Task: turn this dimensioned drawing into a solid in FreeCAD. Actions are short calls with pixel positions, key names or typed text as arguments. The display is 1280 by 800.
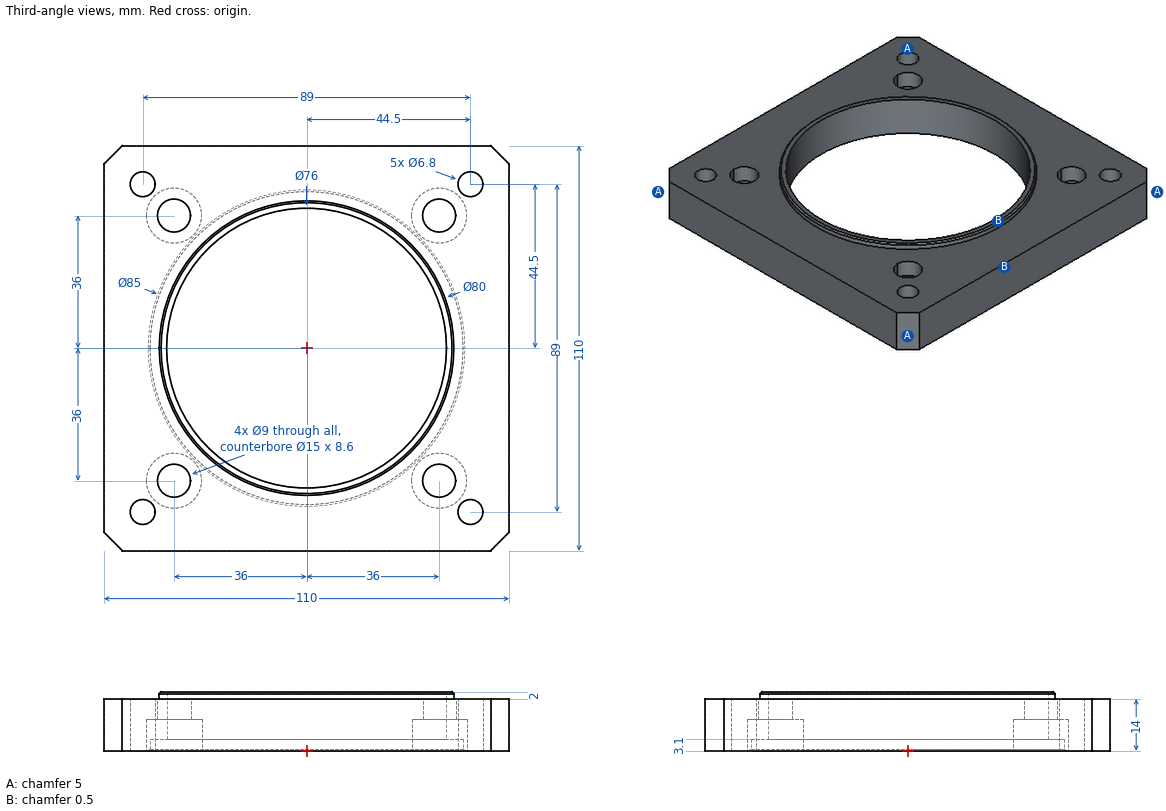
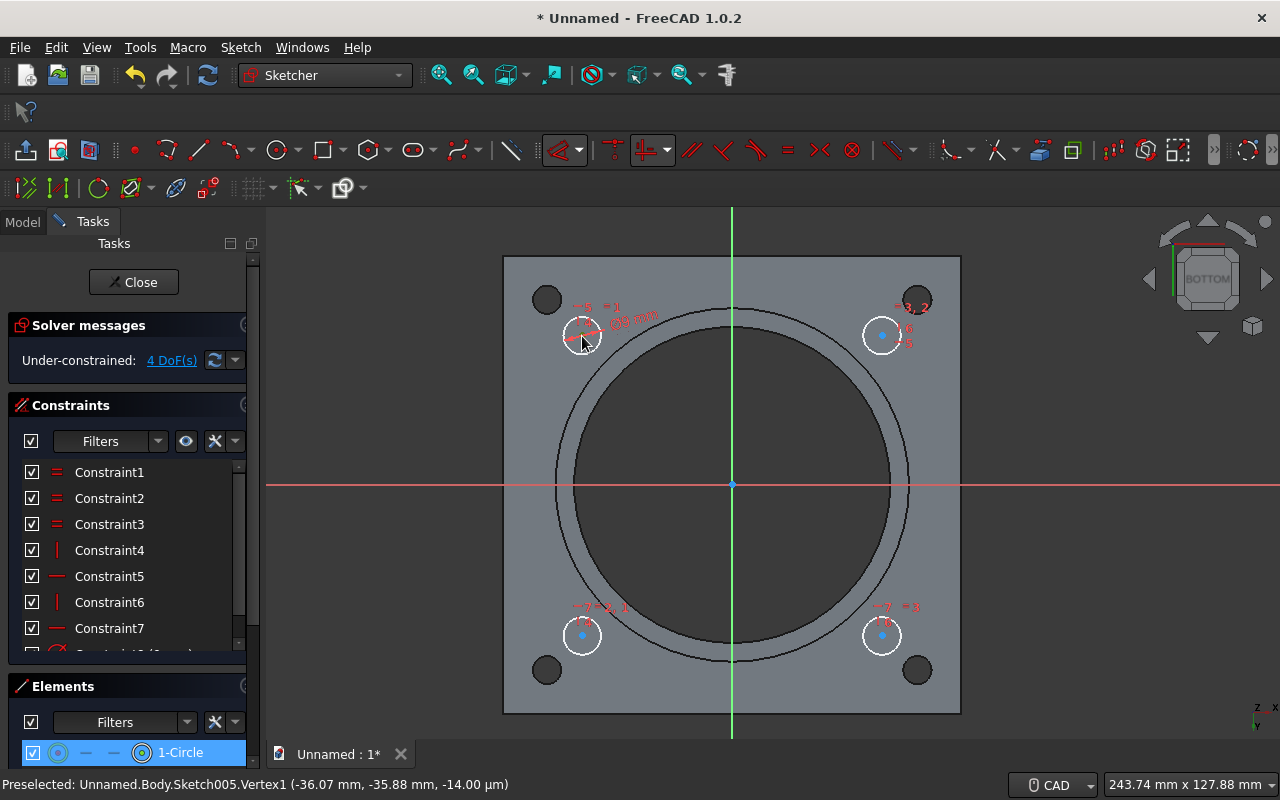
click(582, 150)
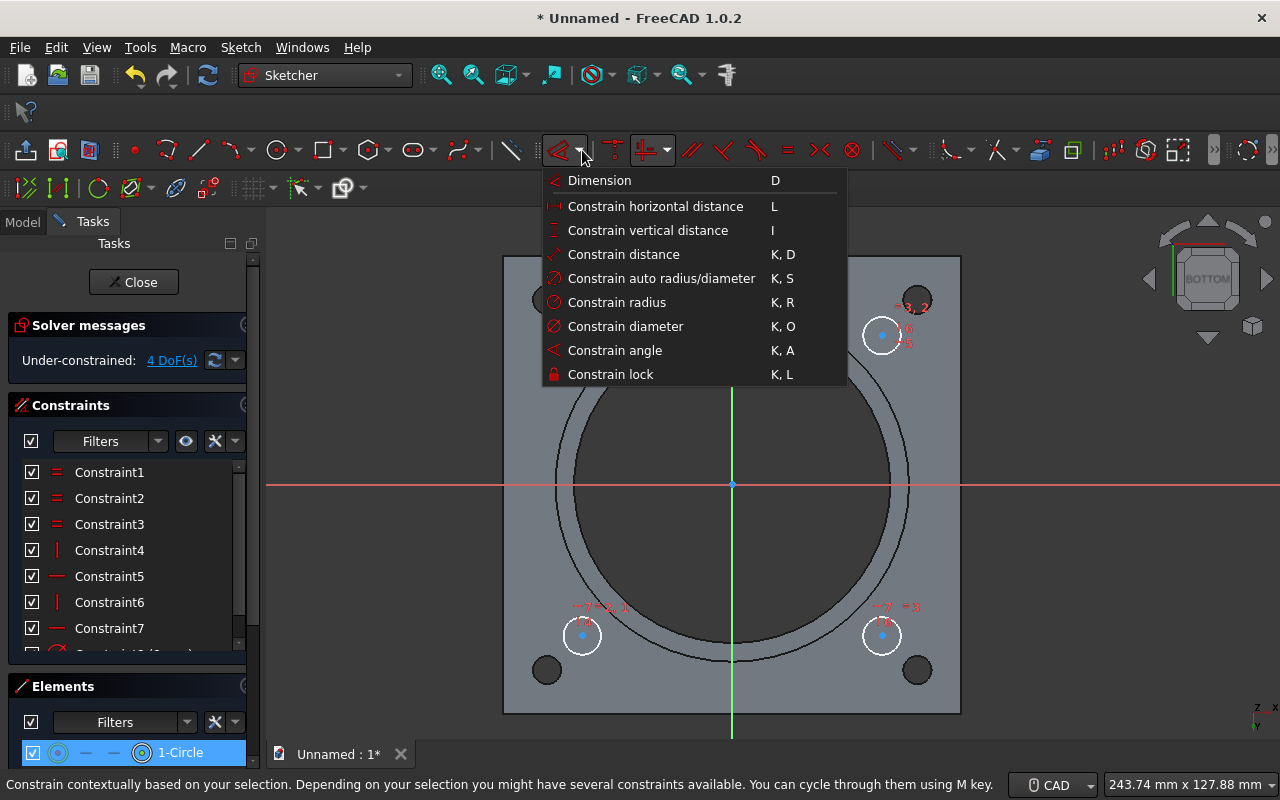
click(695, 206)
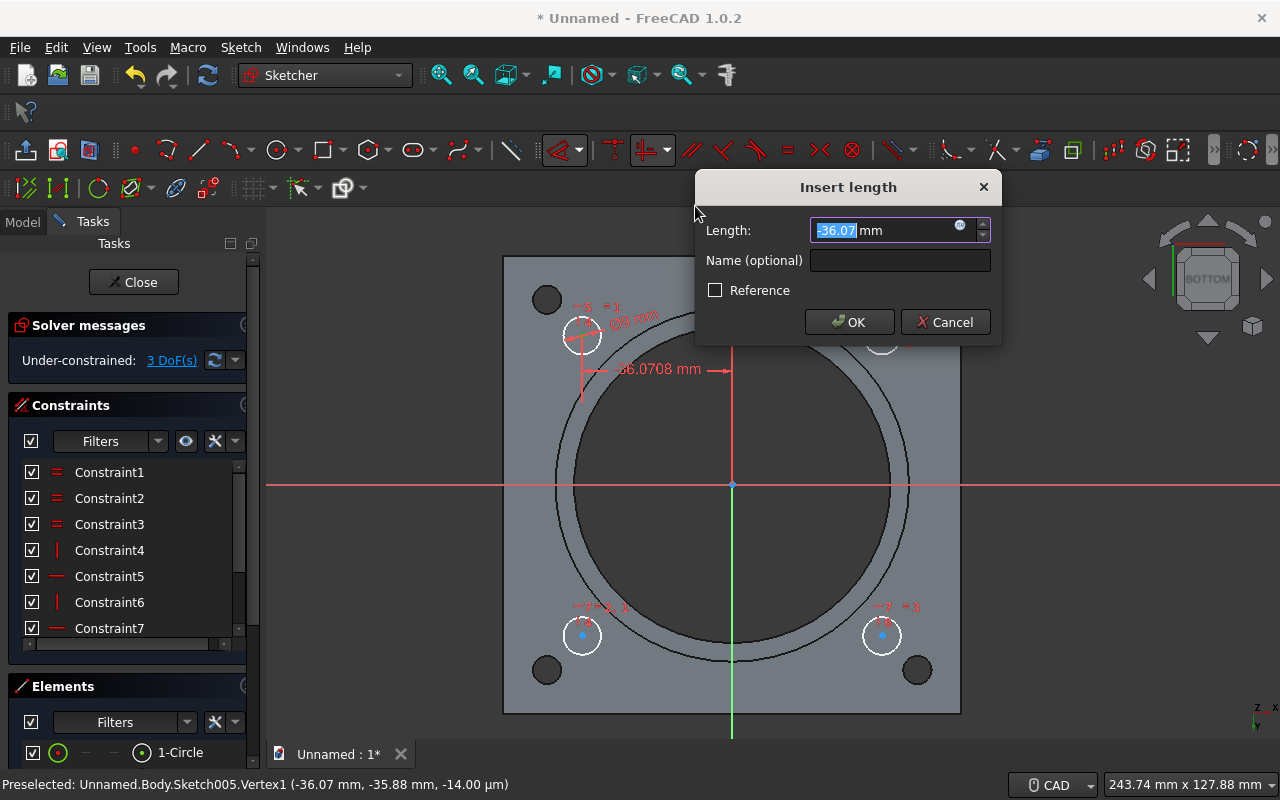
text(-36)
key(Return)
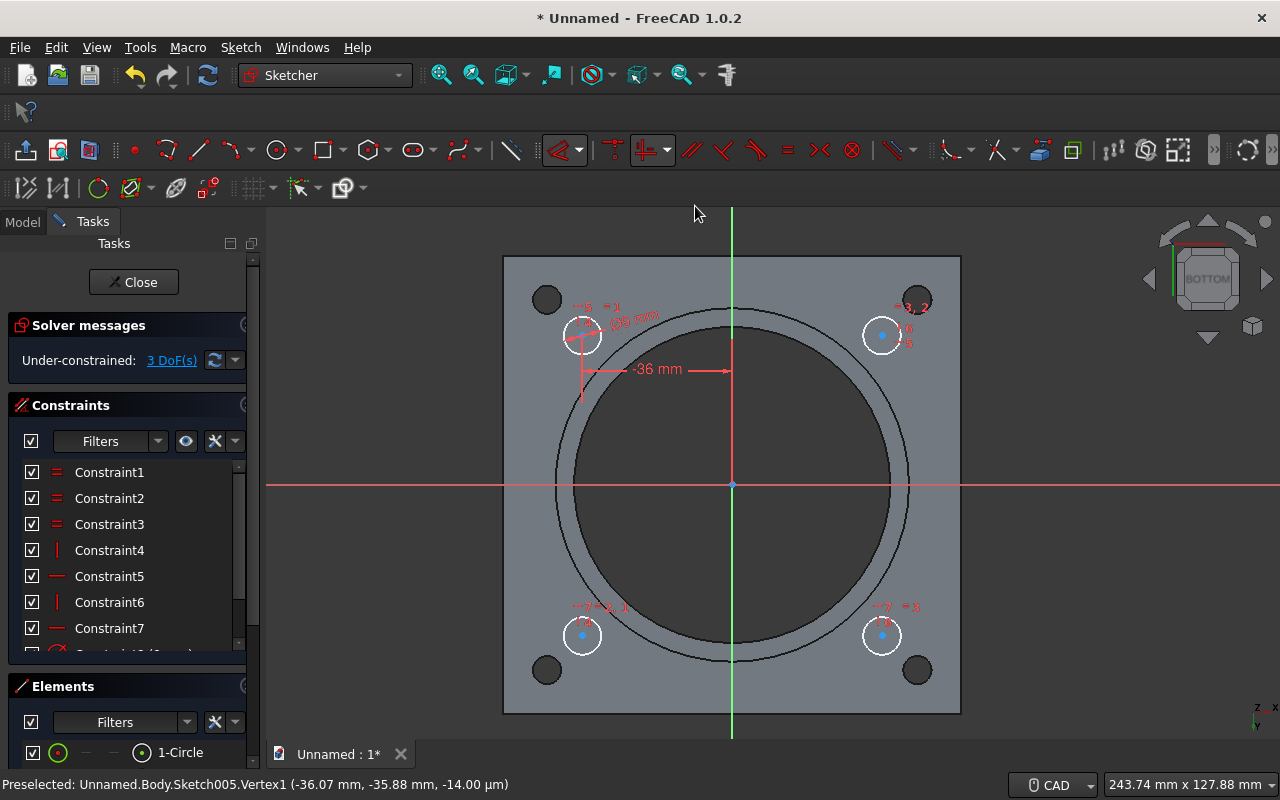
click(582, 336)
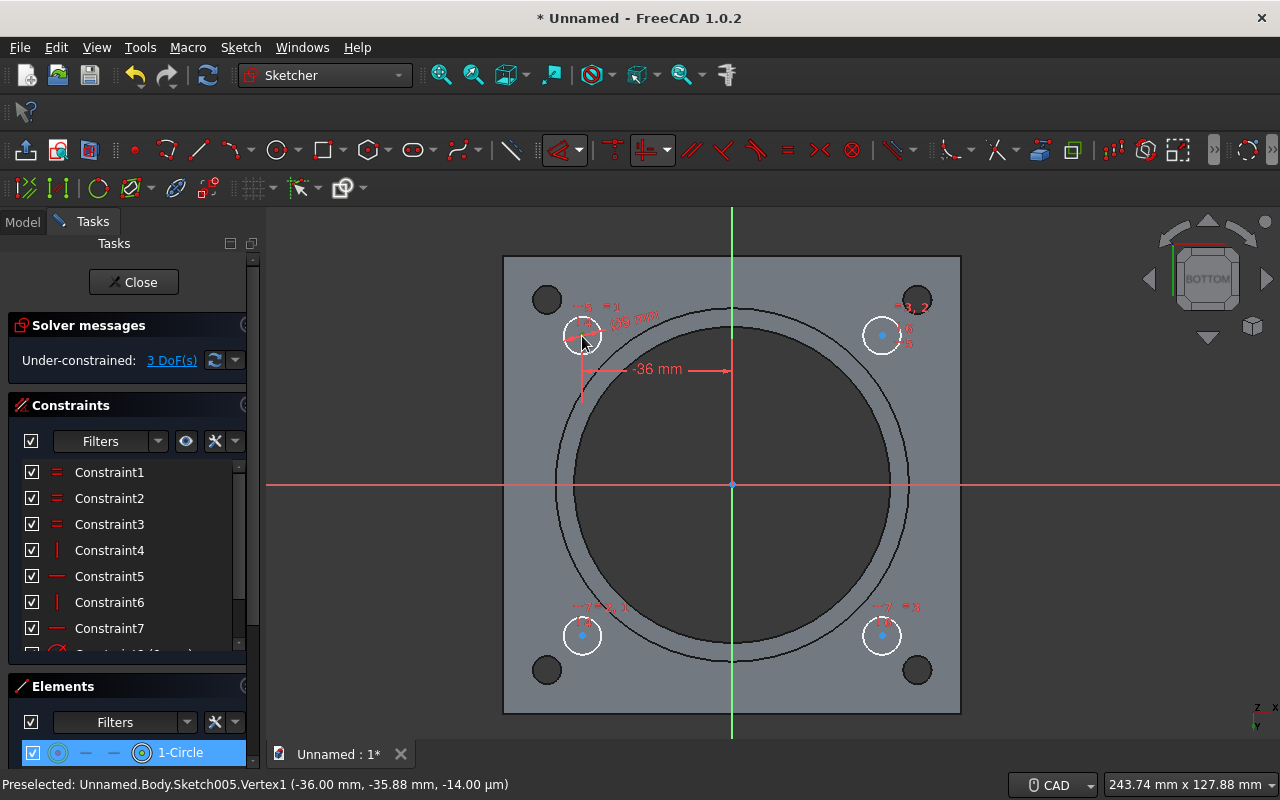
click(582, 150)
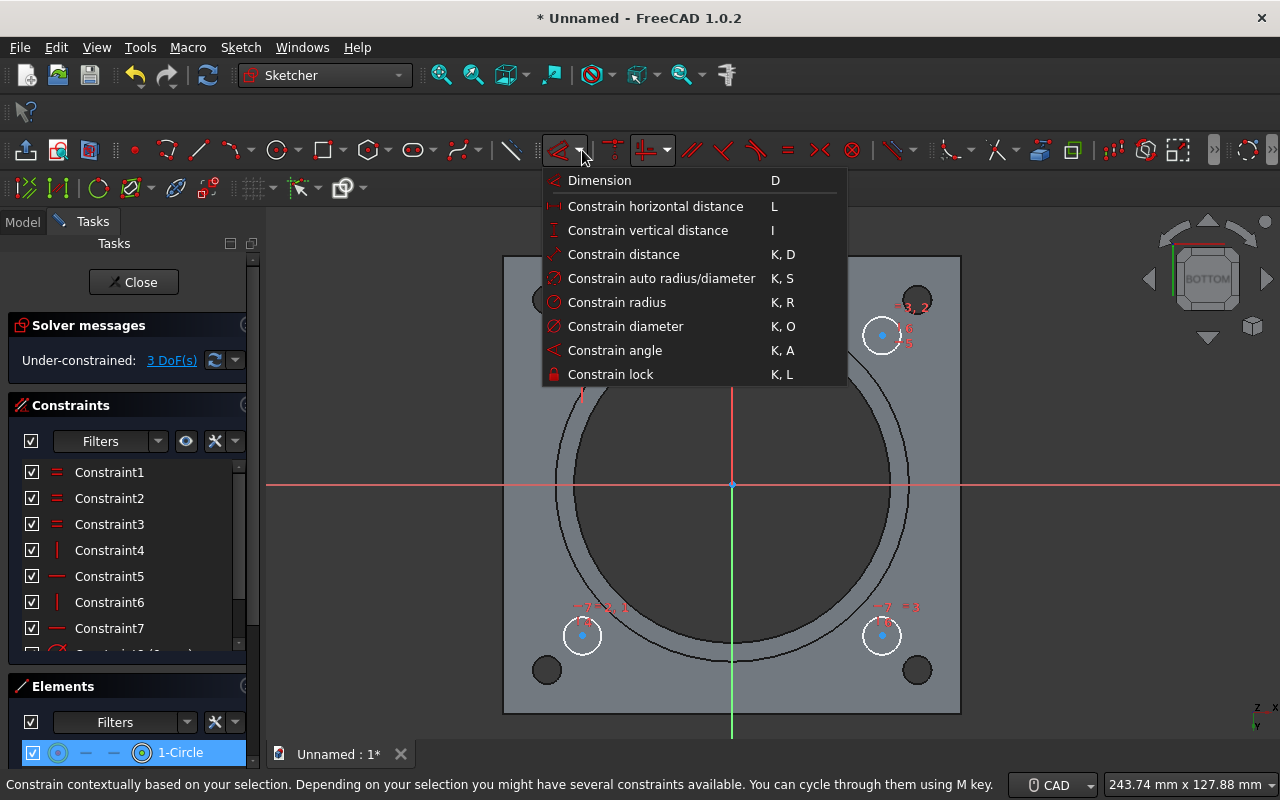
click(695, 230)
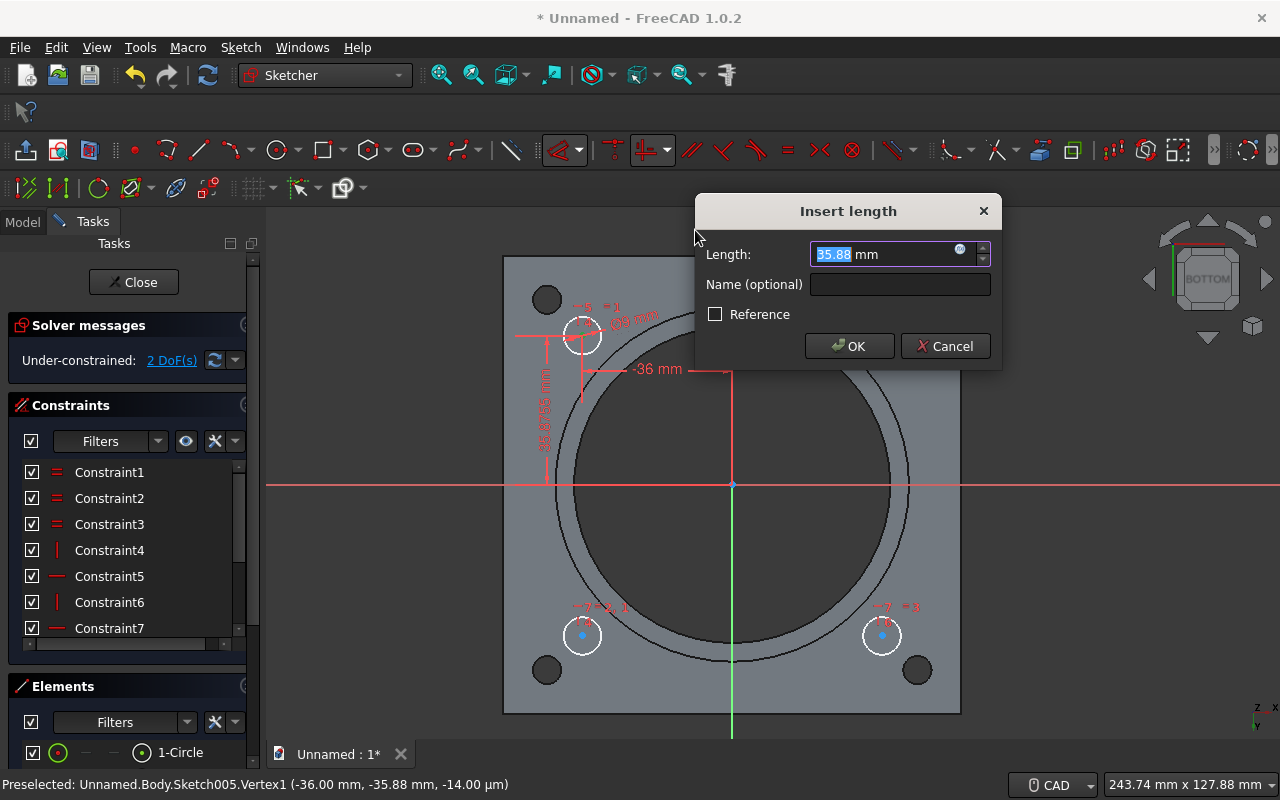
text(36)
key(Return)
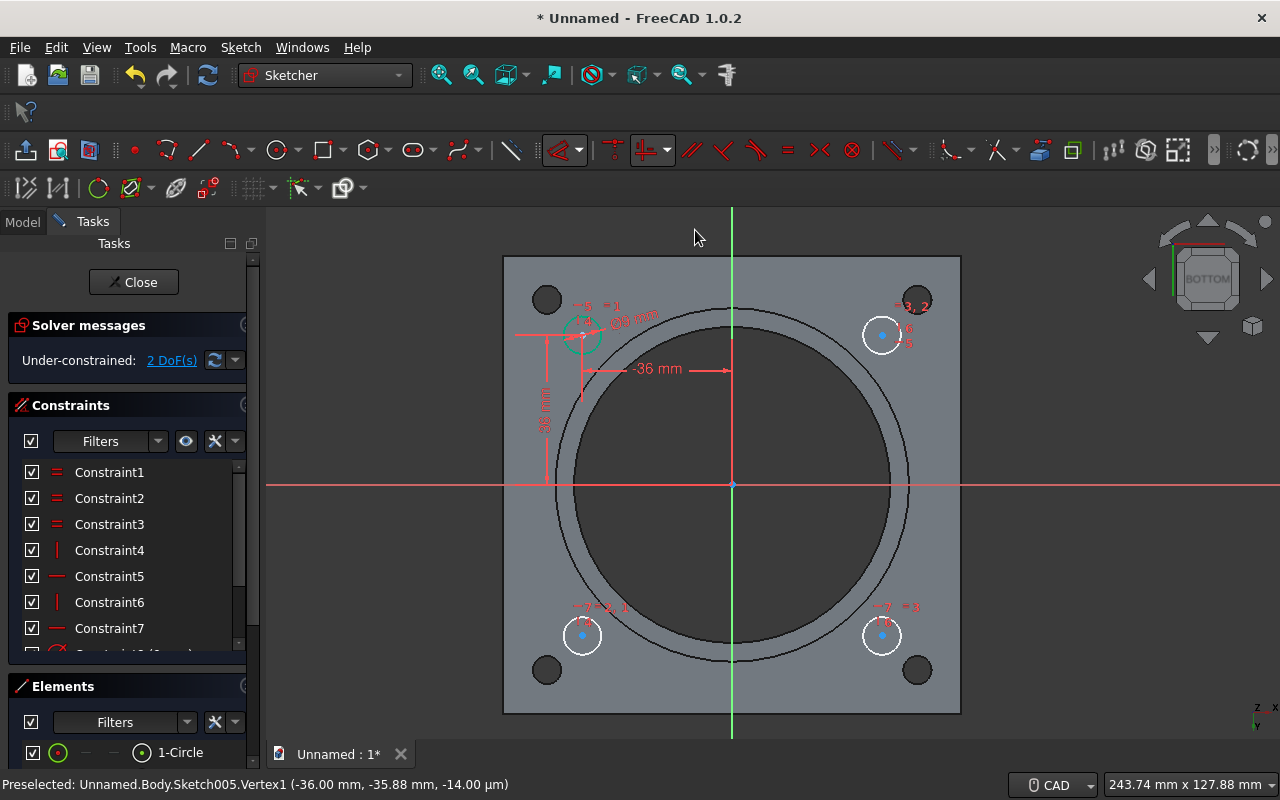
click(582, 636)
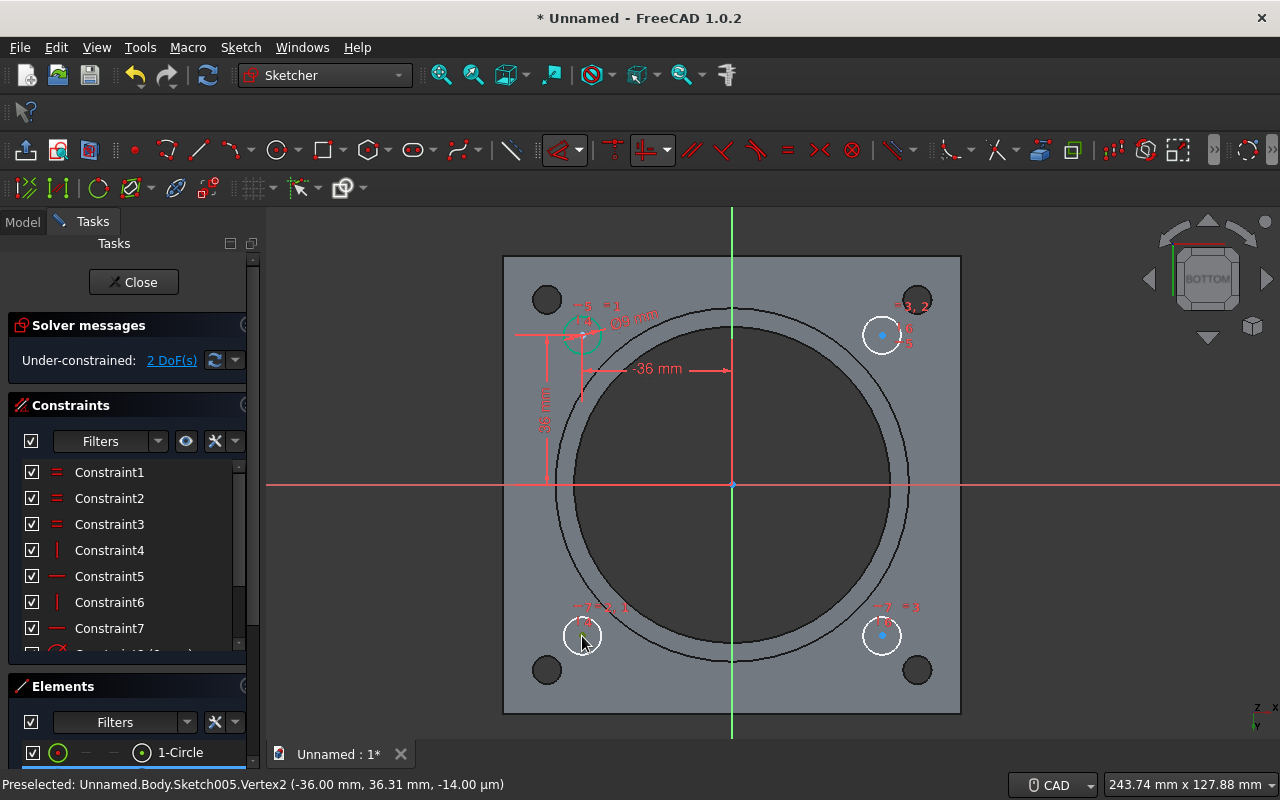
key(i)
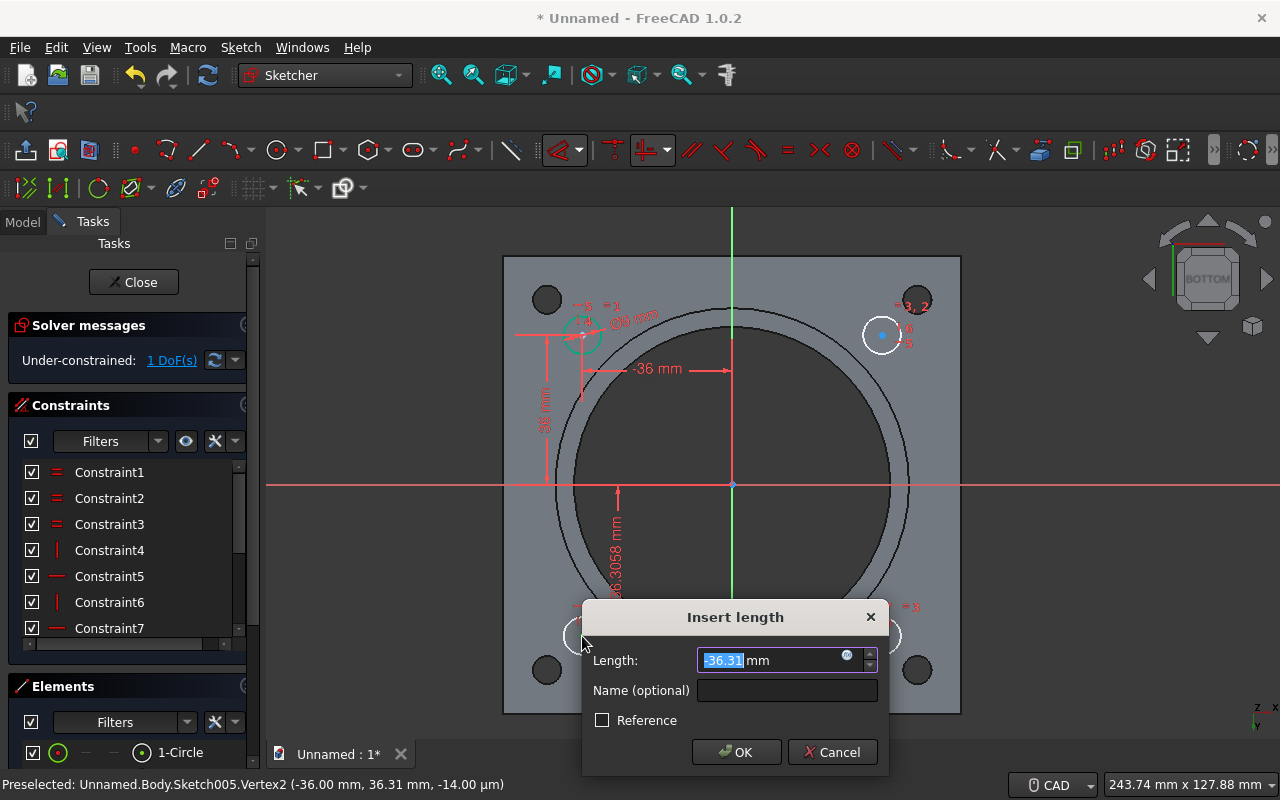
text(-36)
key(Return)